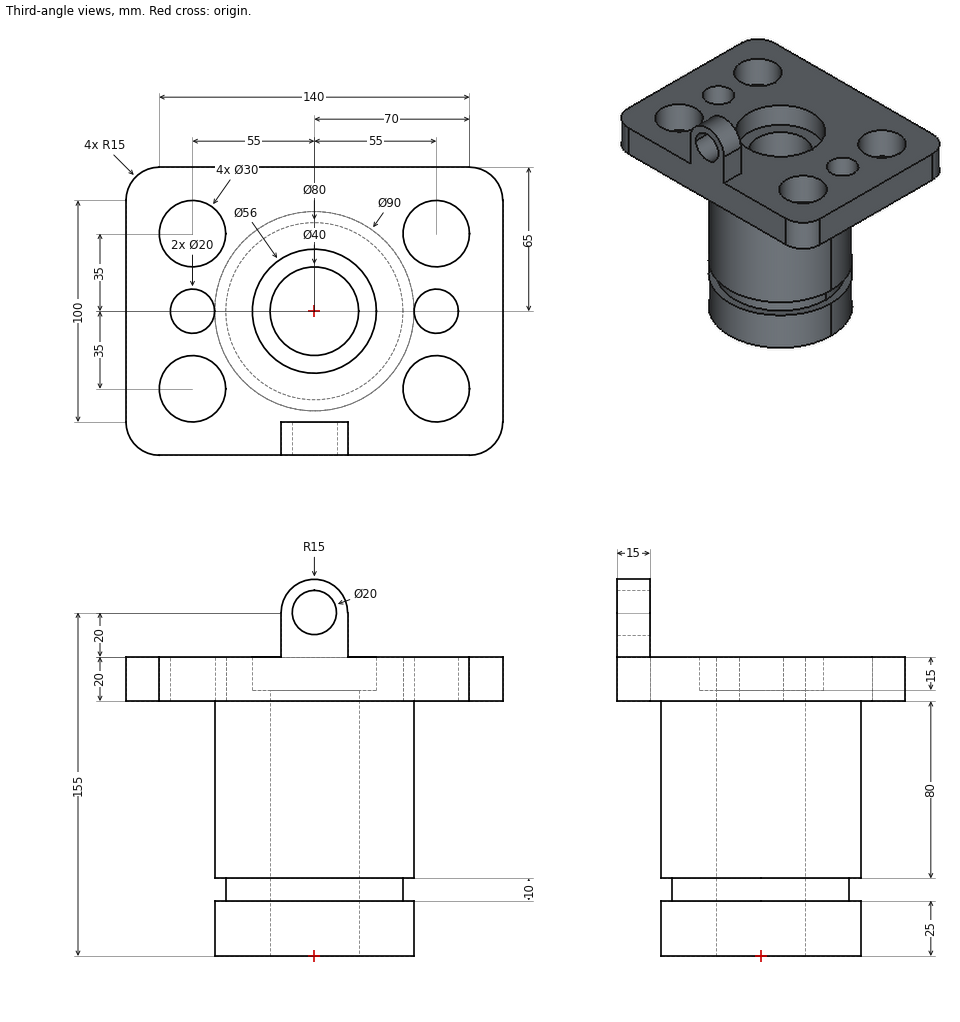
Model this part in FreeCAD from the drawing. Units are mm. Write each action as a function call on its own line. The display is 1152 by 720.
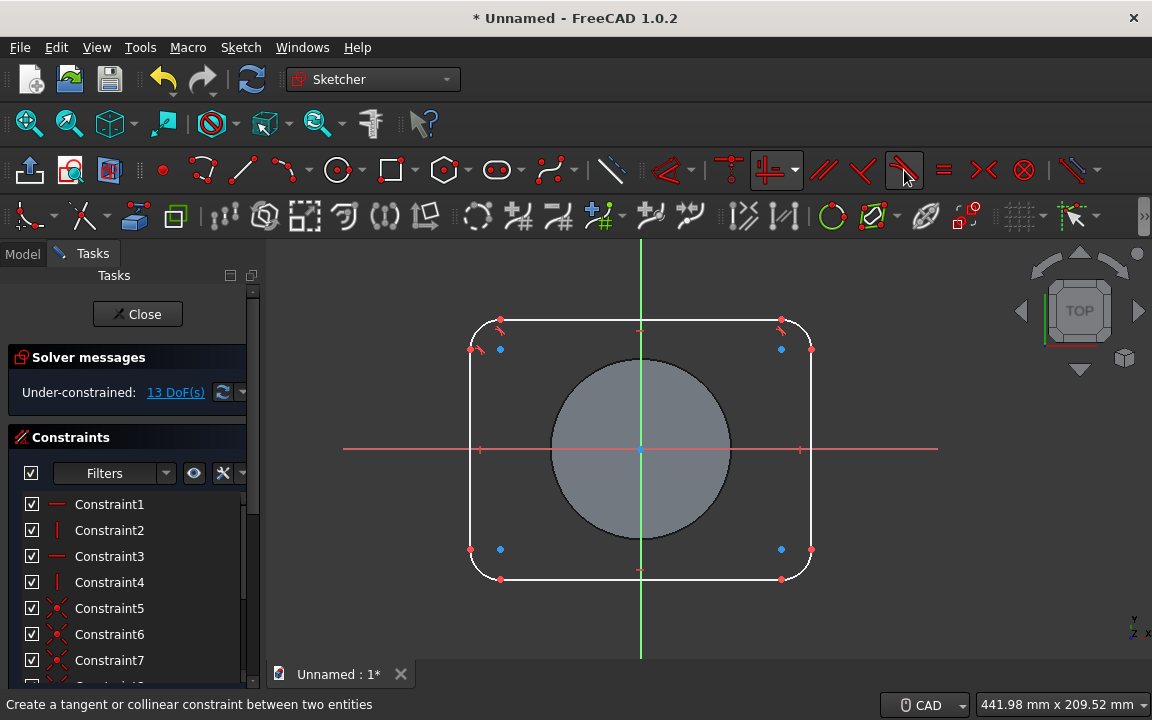
click(470, 410)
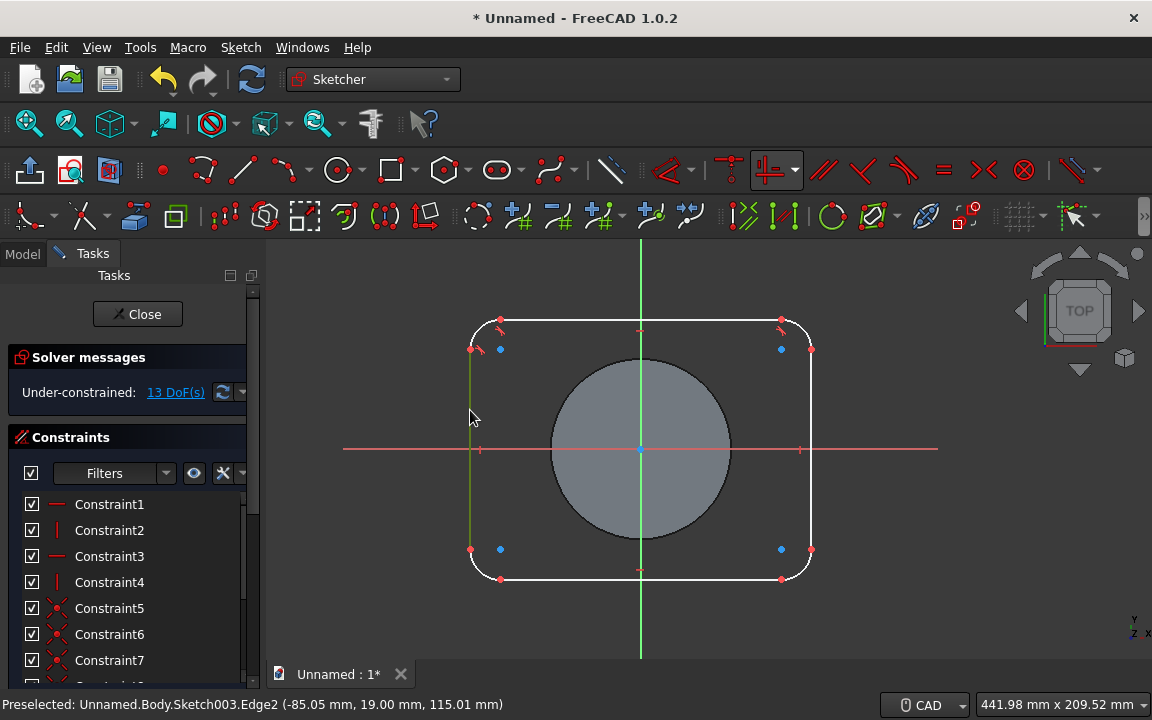
click(474, 564)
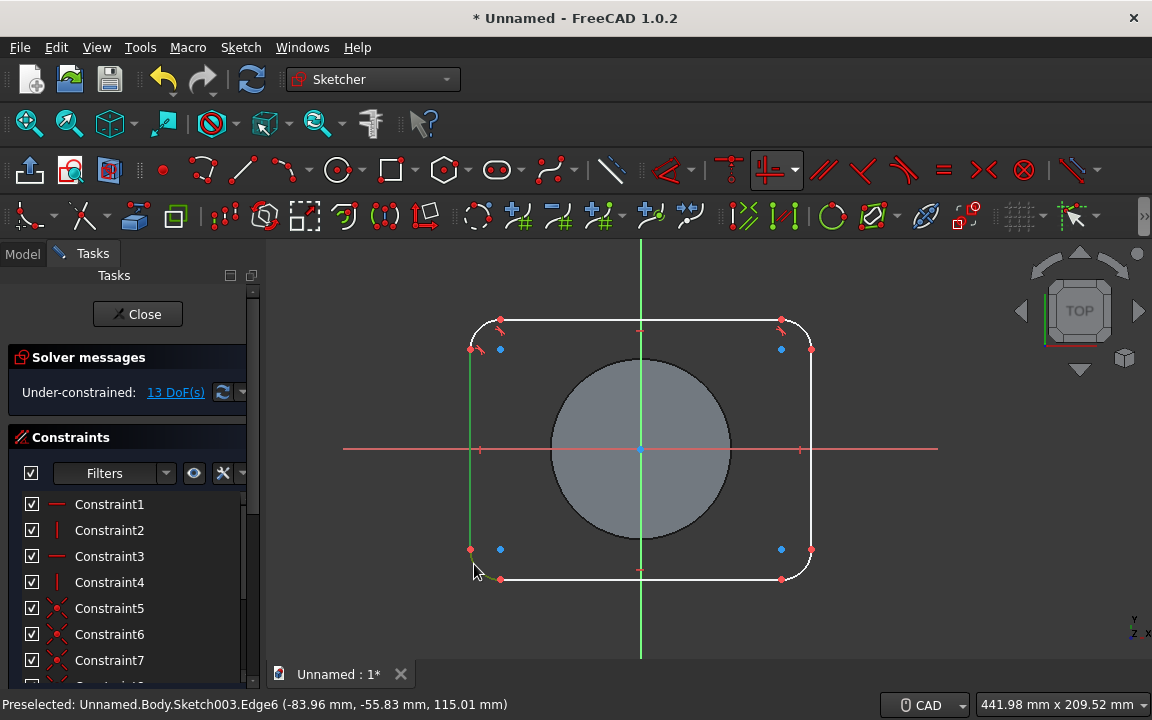
click(904, 170)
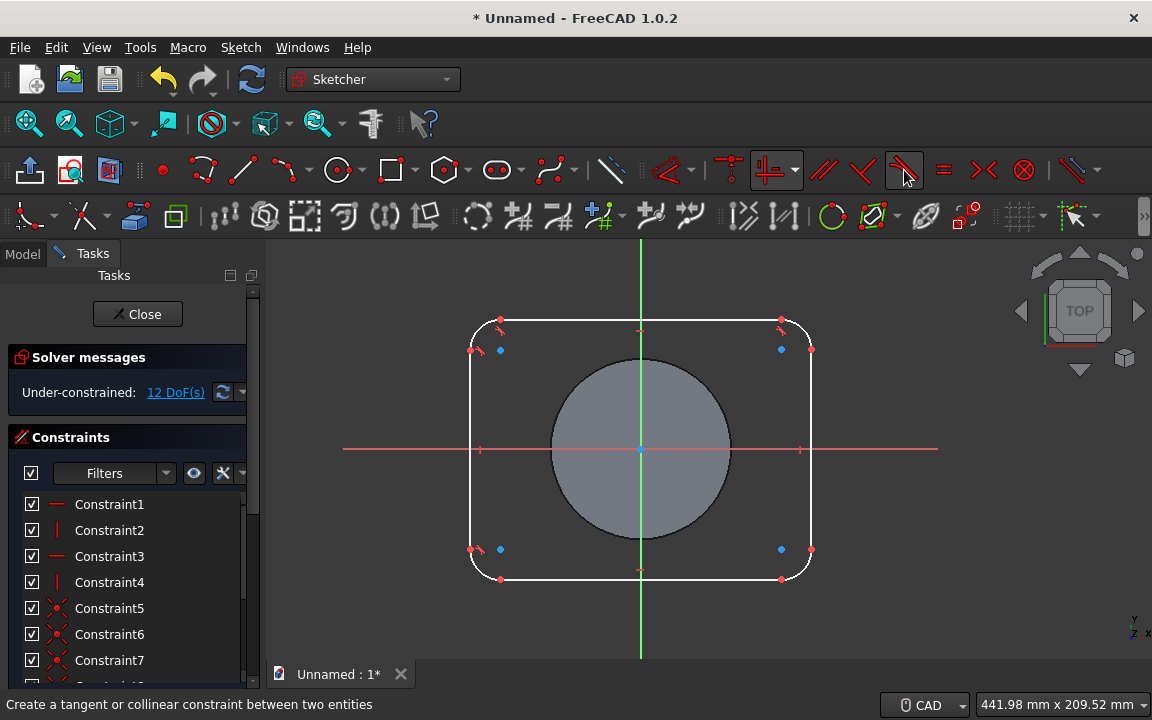
click(585, 580)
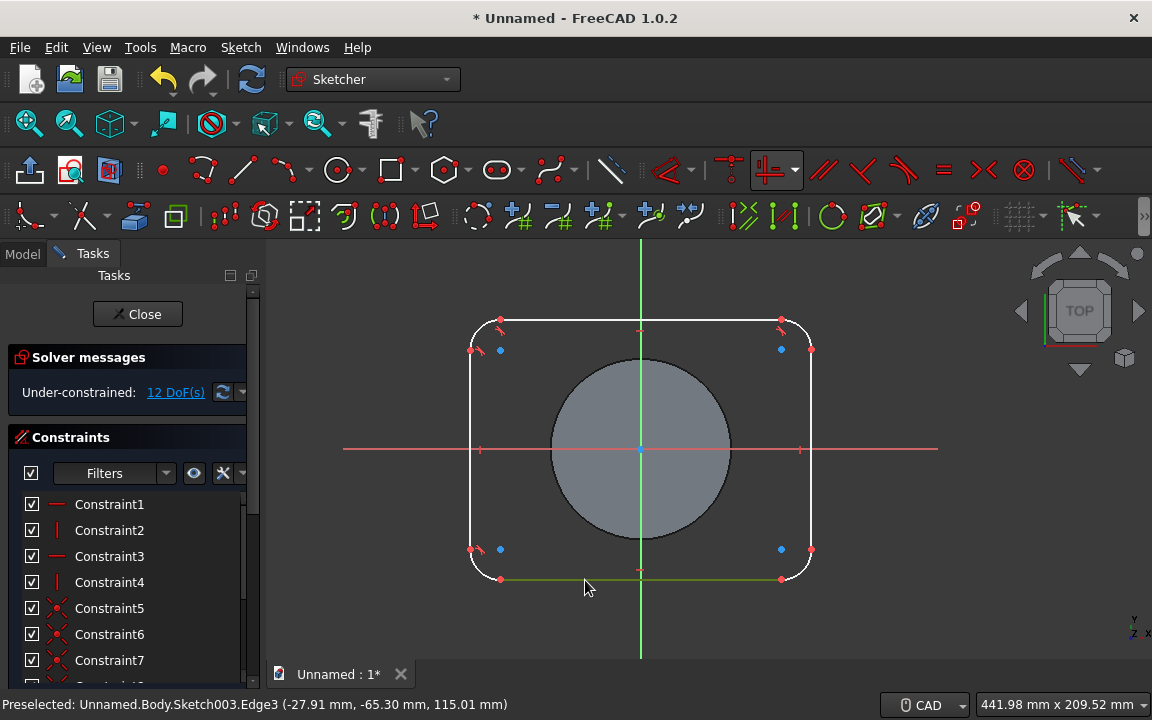
click(474, 563)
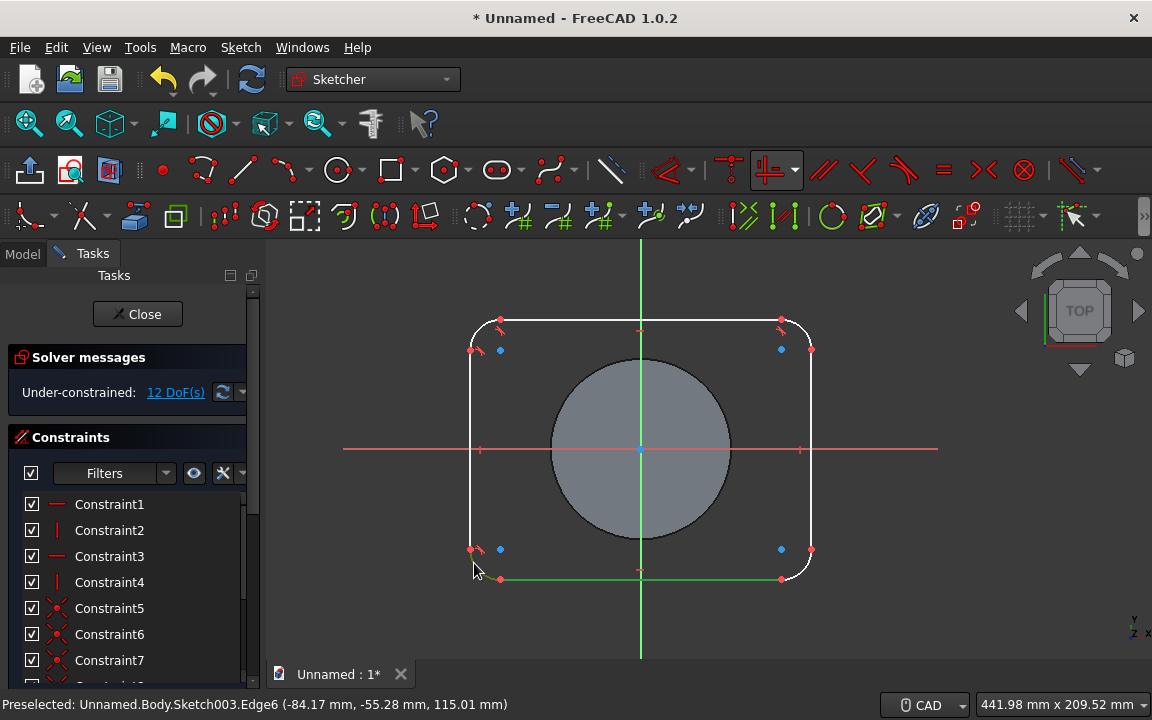
click(904, 170)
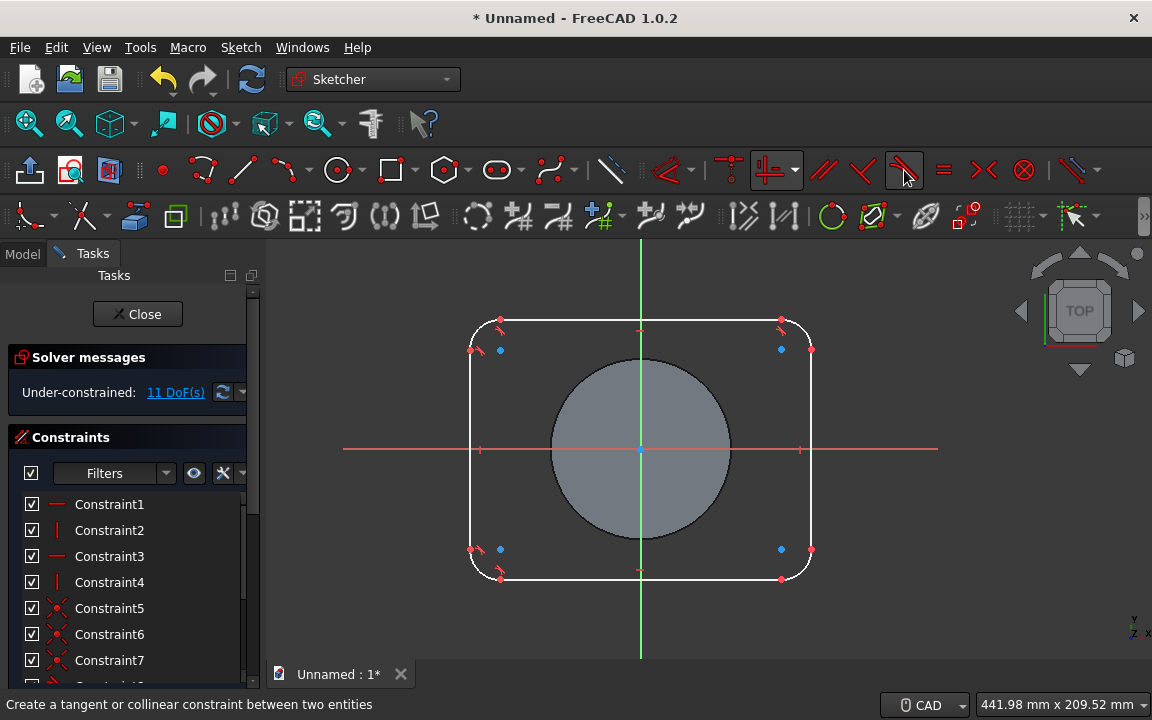
click(585, 580)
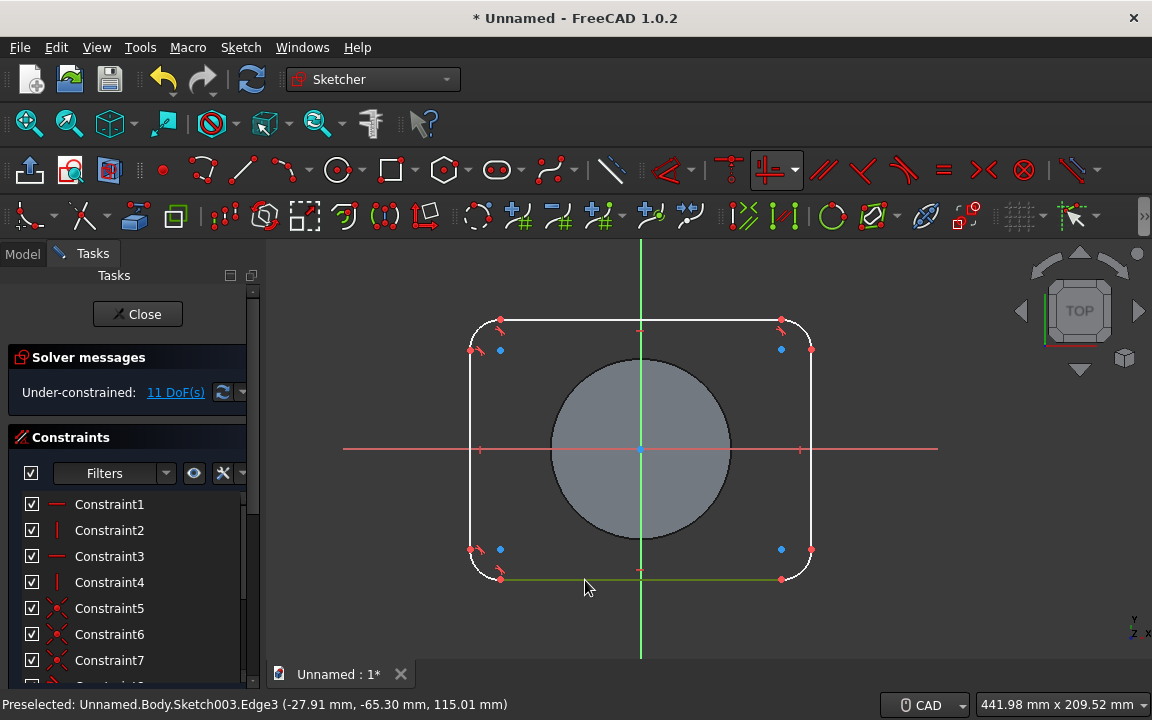
click(795, 577)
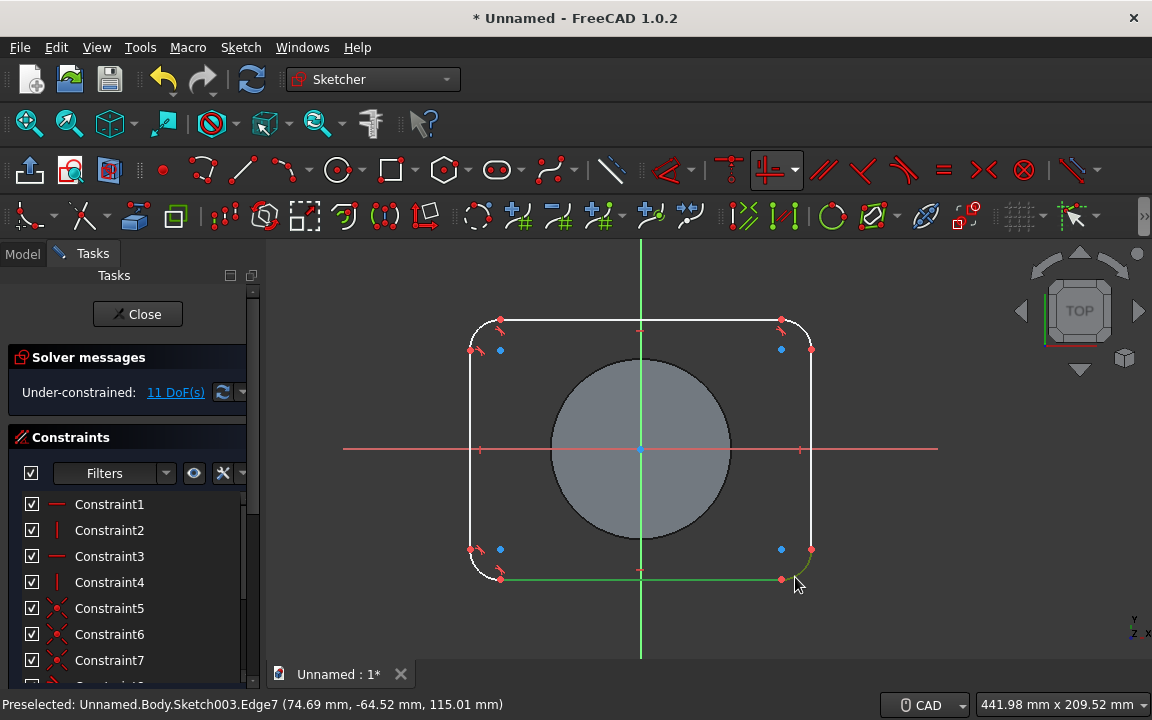
click(904, 170)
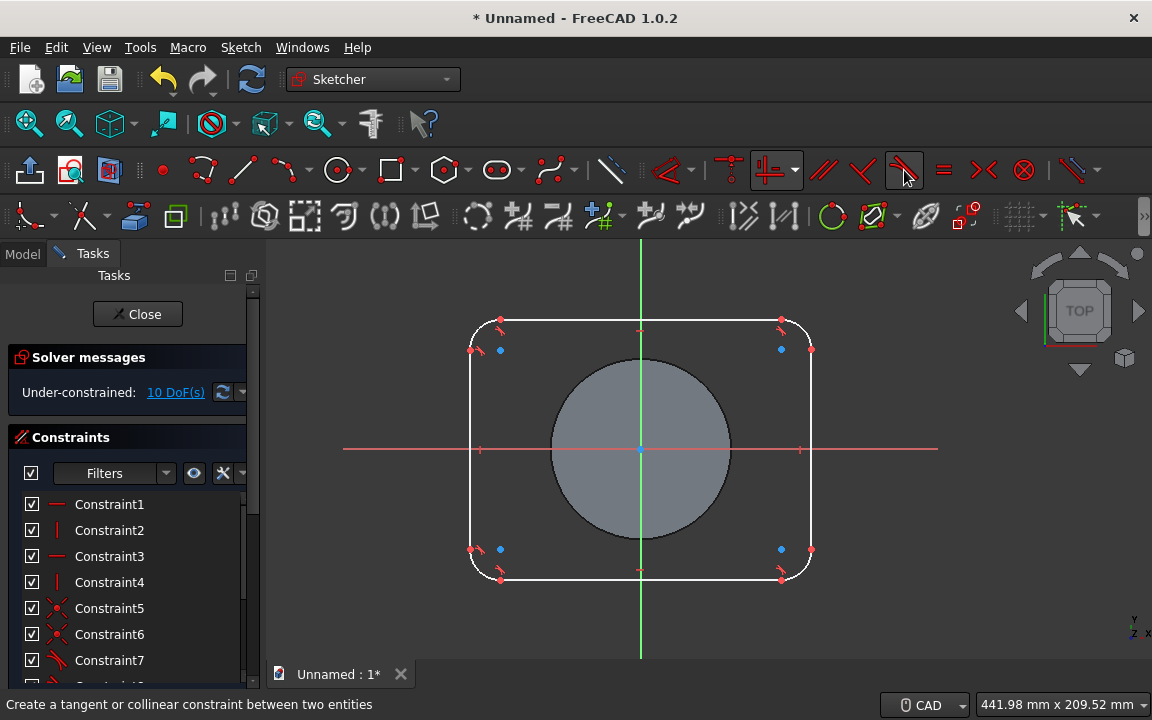
click(811, 490)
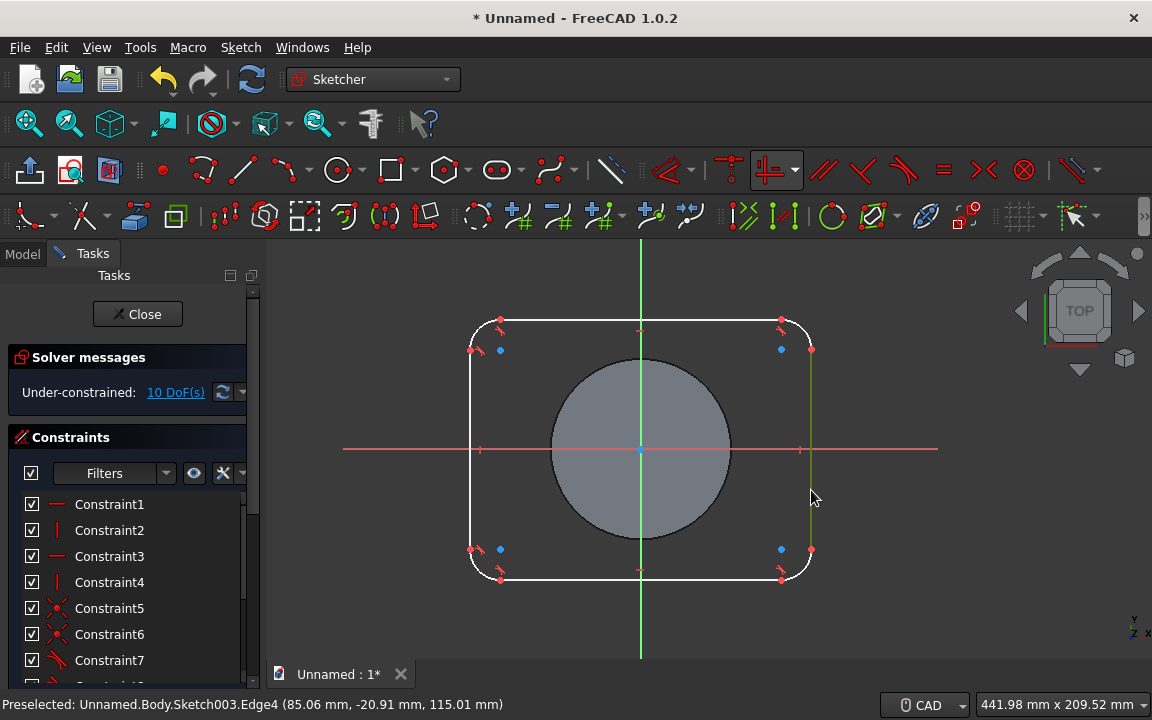
click(795, 577)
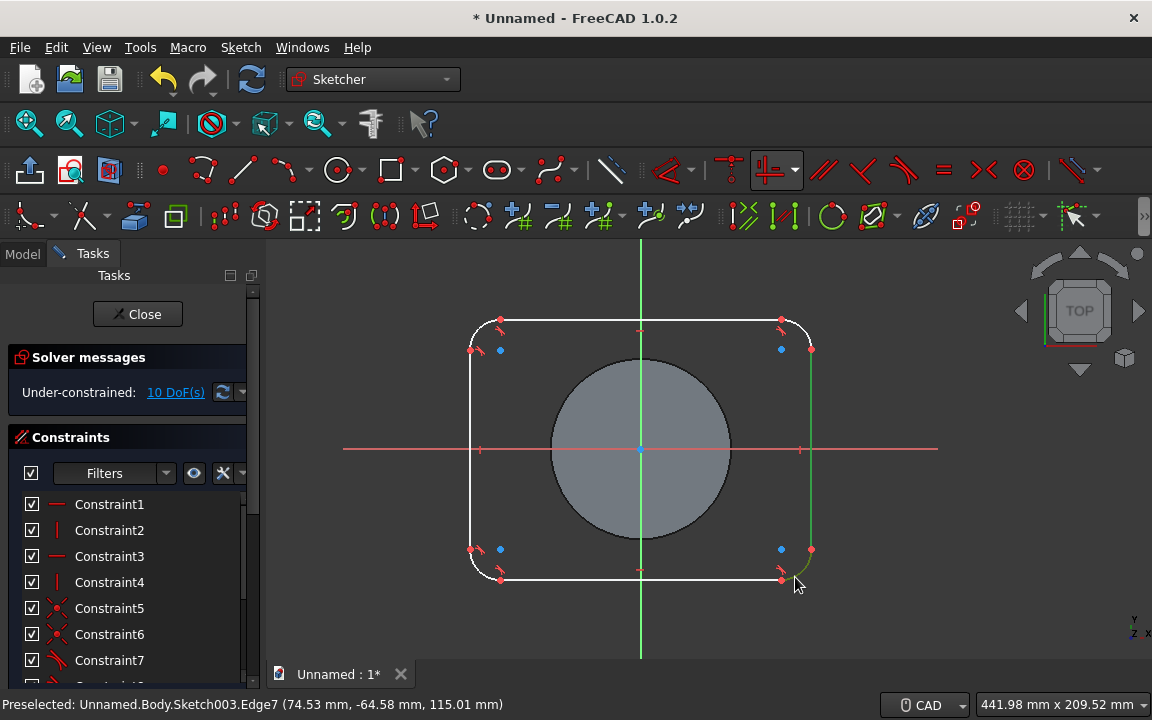
click(904, 170)